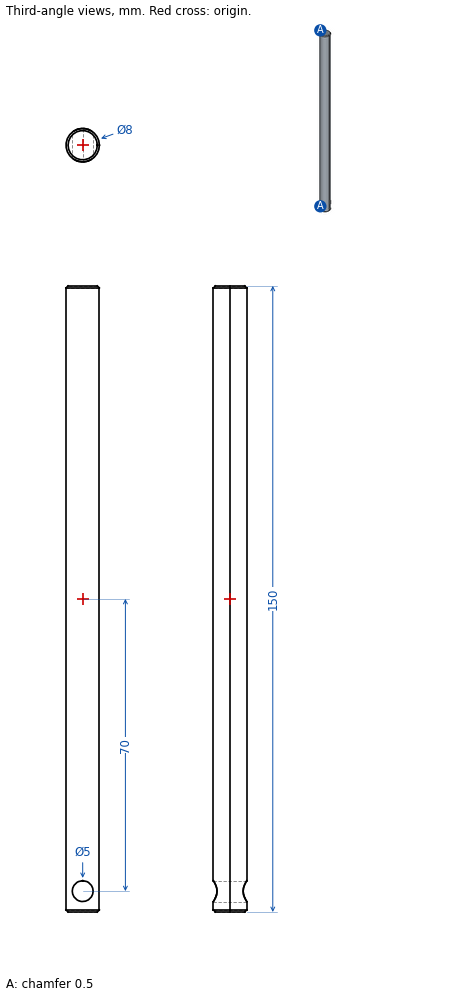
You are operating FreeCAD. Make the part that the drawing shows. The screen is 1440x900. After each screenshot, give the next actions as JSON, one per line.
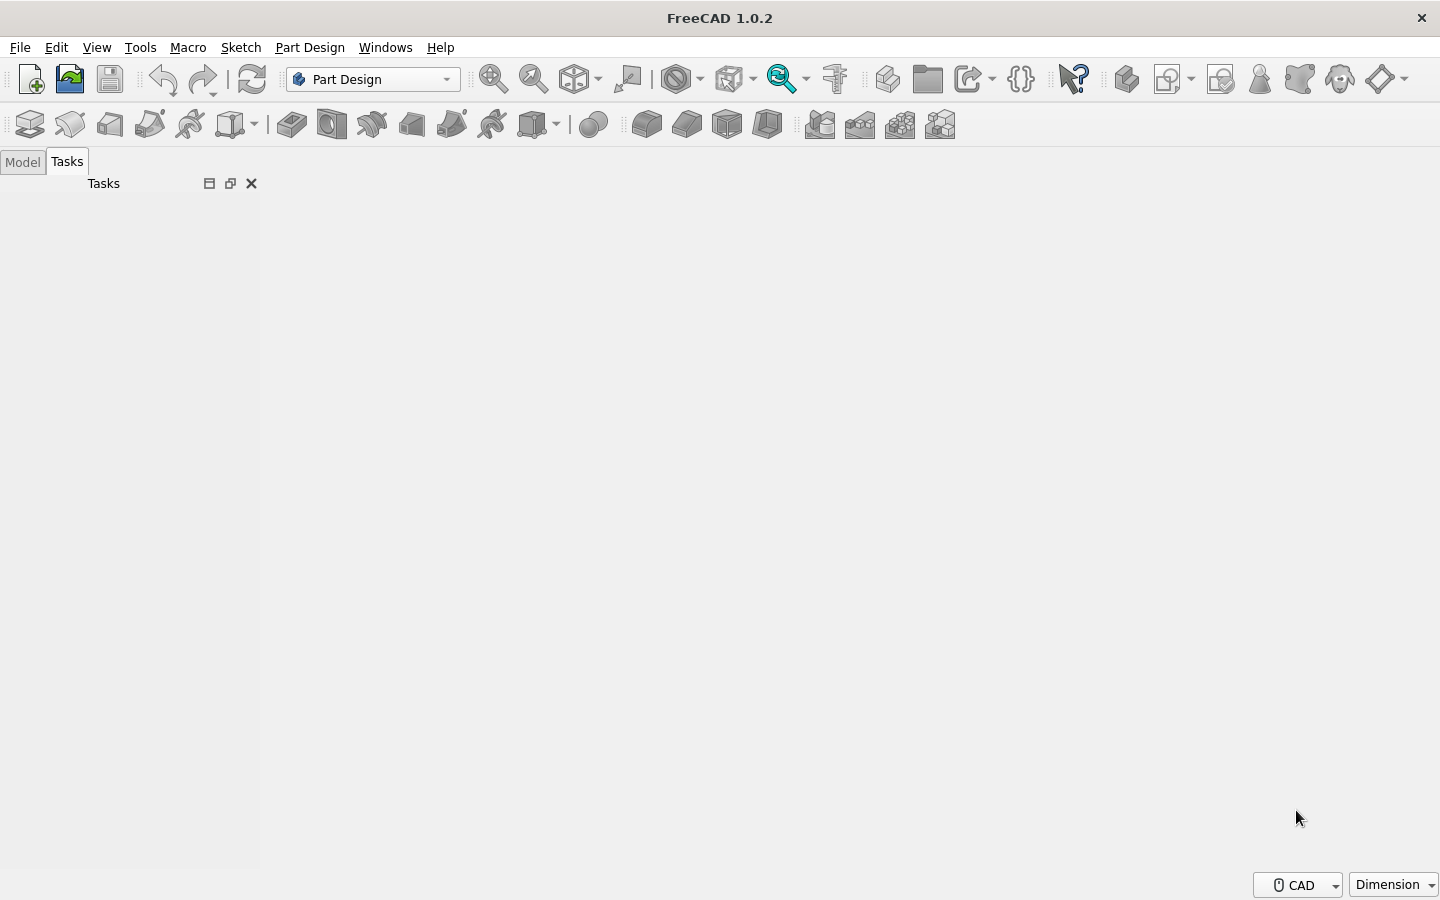
{"action": "key", "text": "ctrl+n"}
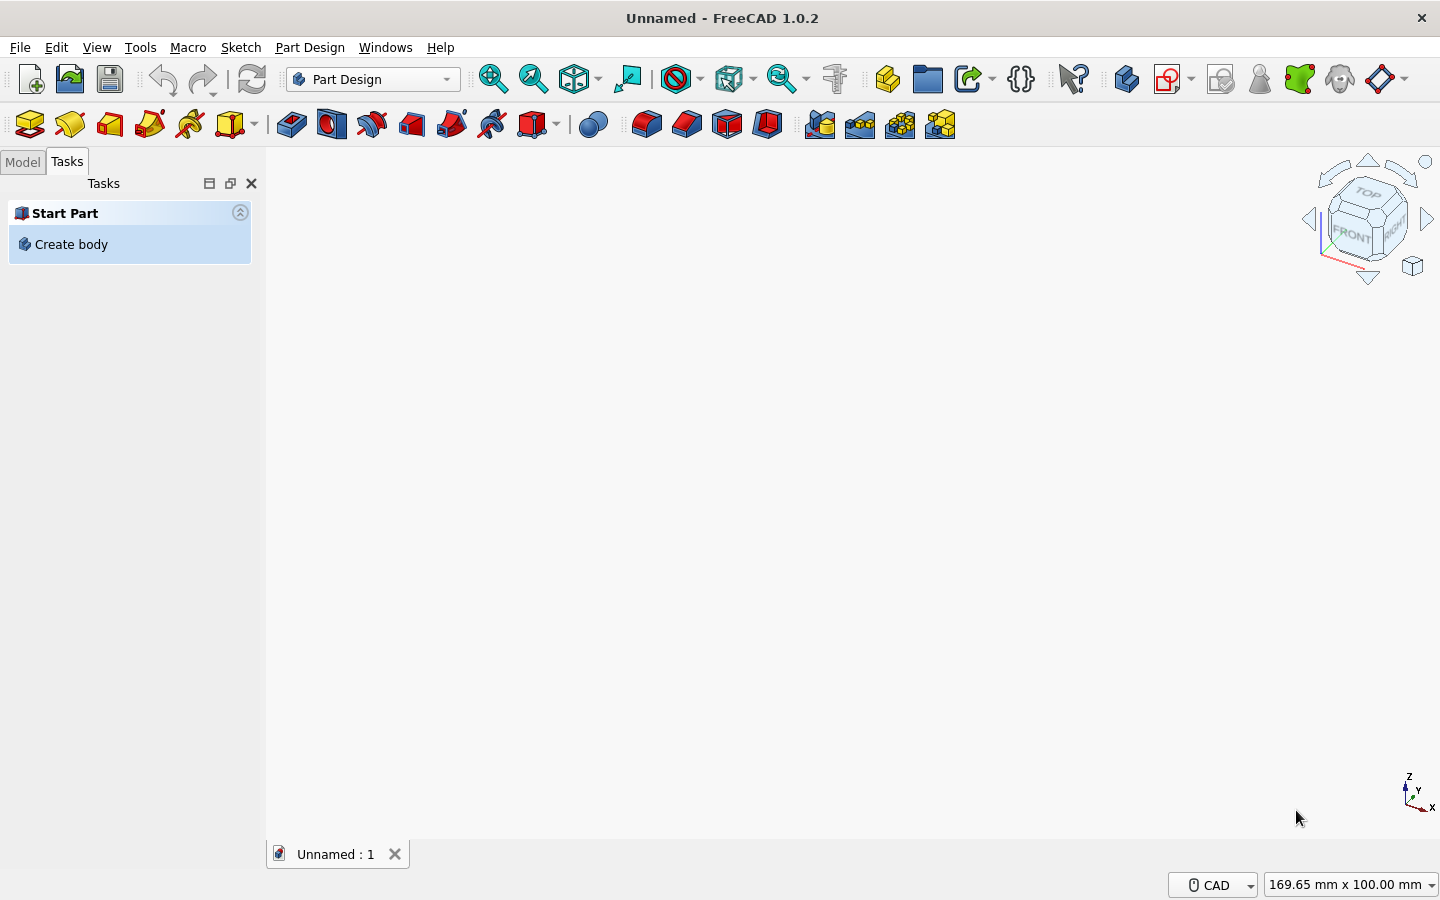
{"action": "left_click", "coordinate": [1168, 80]}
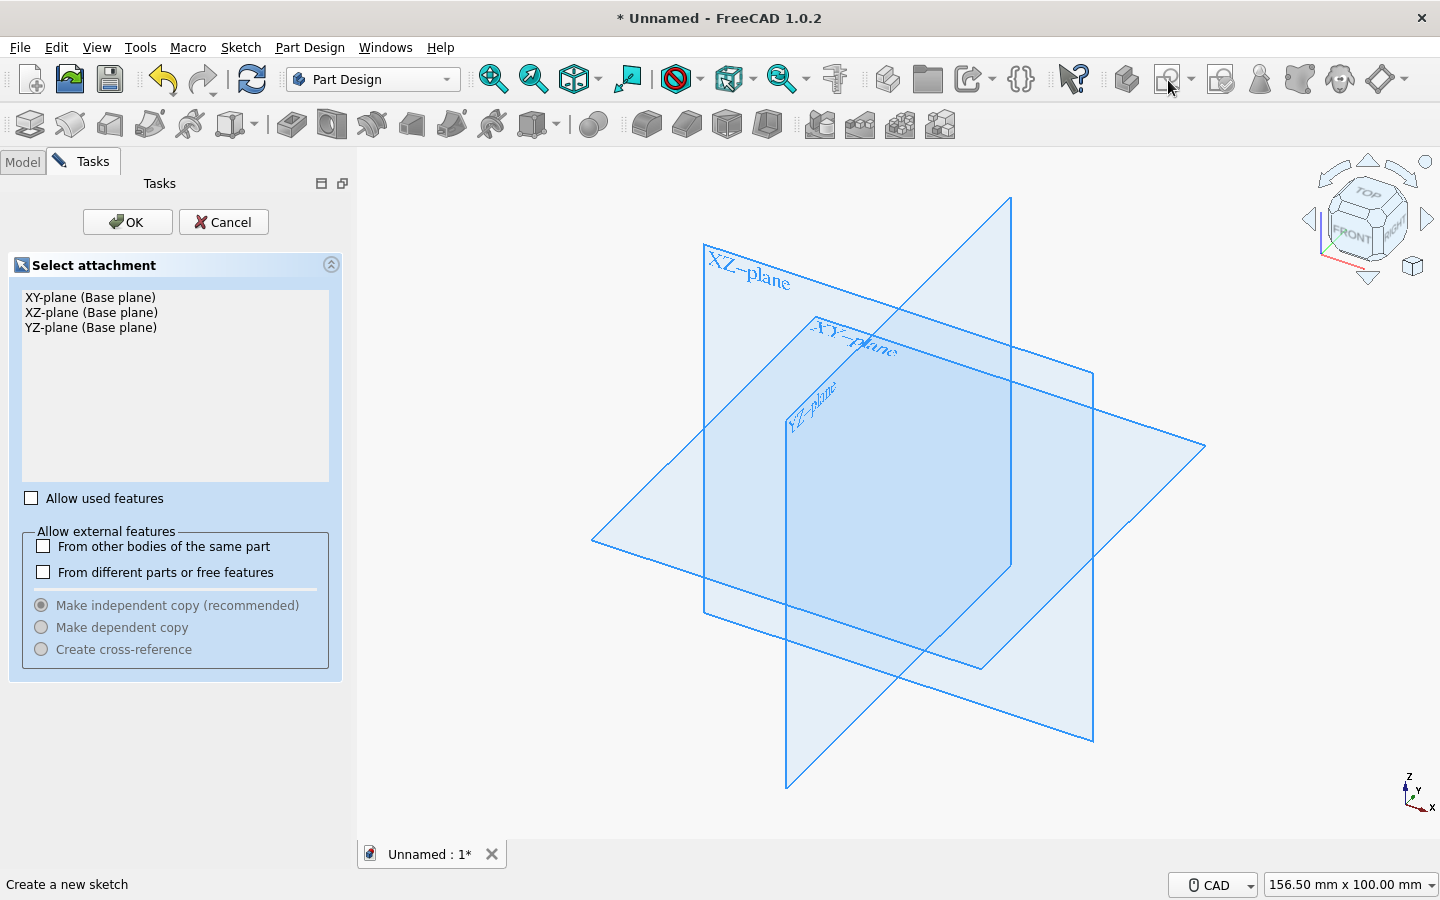
{"action": "left_click", "coordinate": [82, 298]}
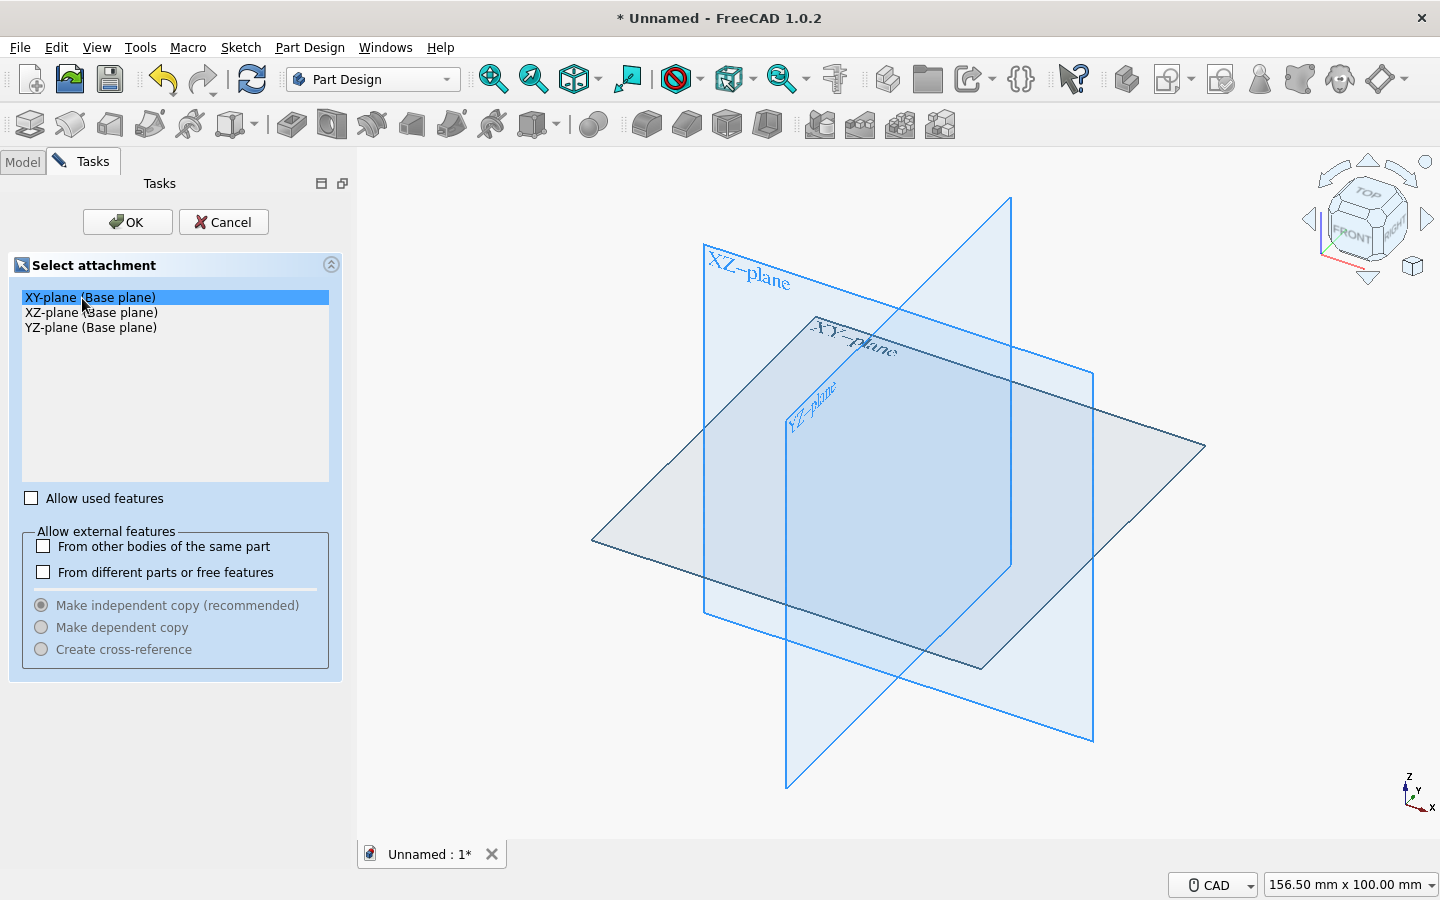
{"action": "left_click", "coordinate": [128, 222]}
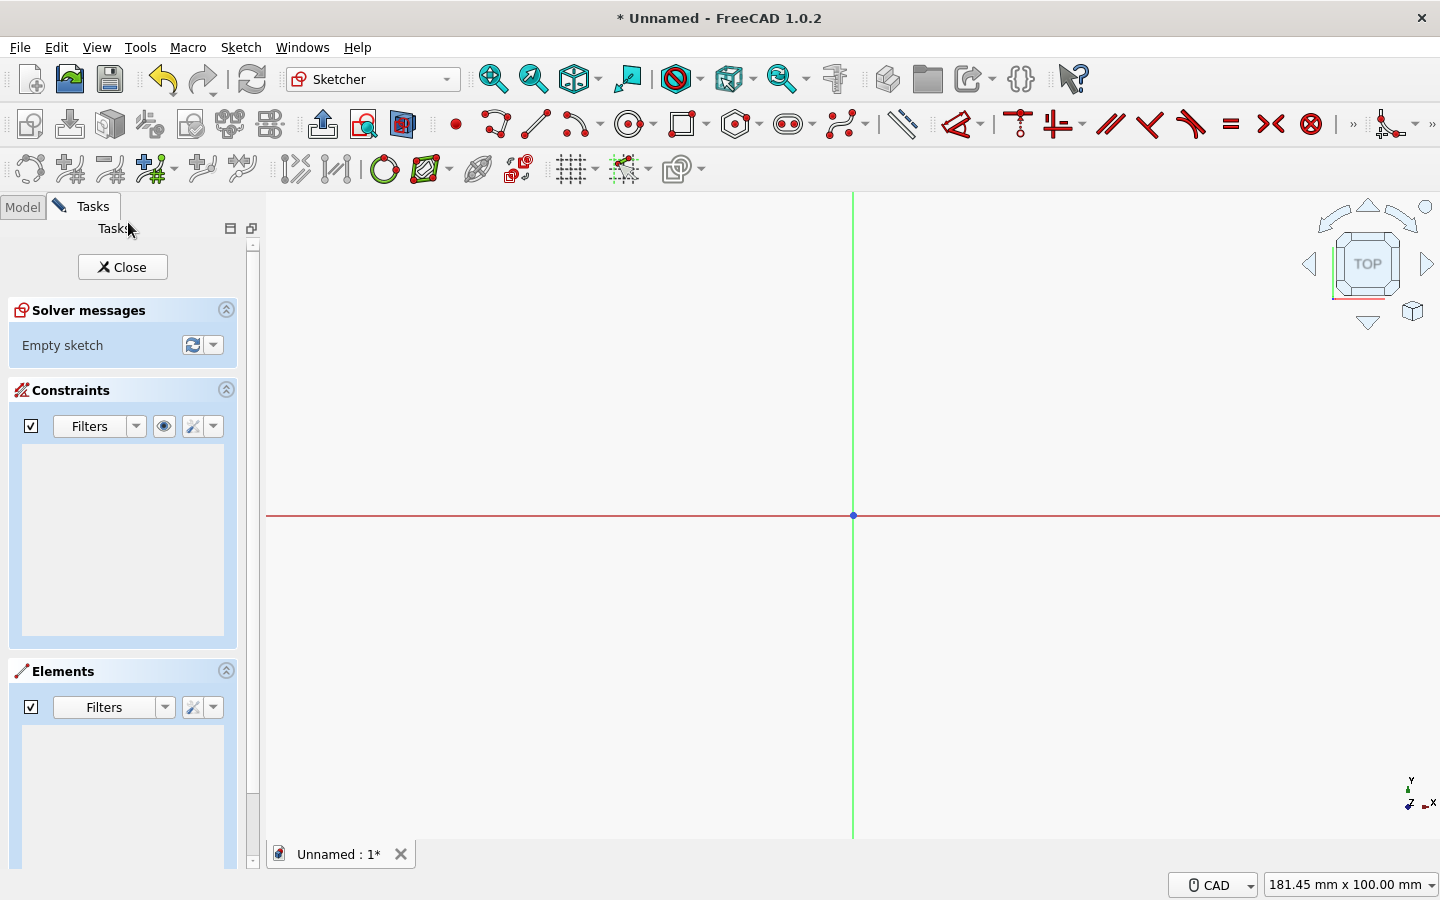
{"action": "scroll", "coordinate": [864, 516], "scroll_direction": "up", "scroll_amount": 10}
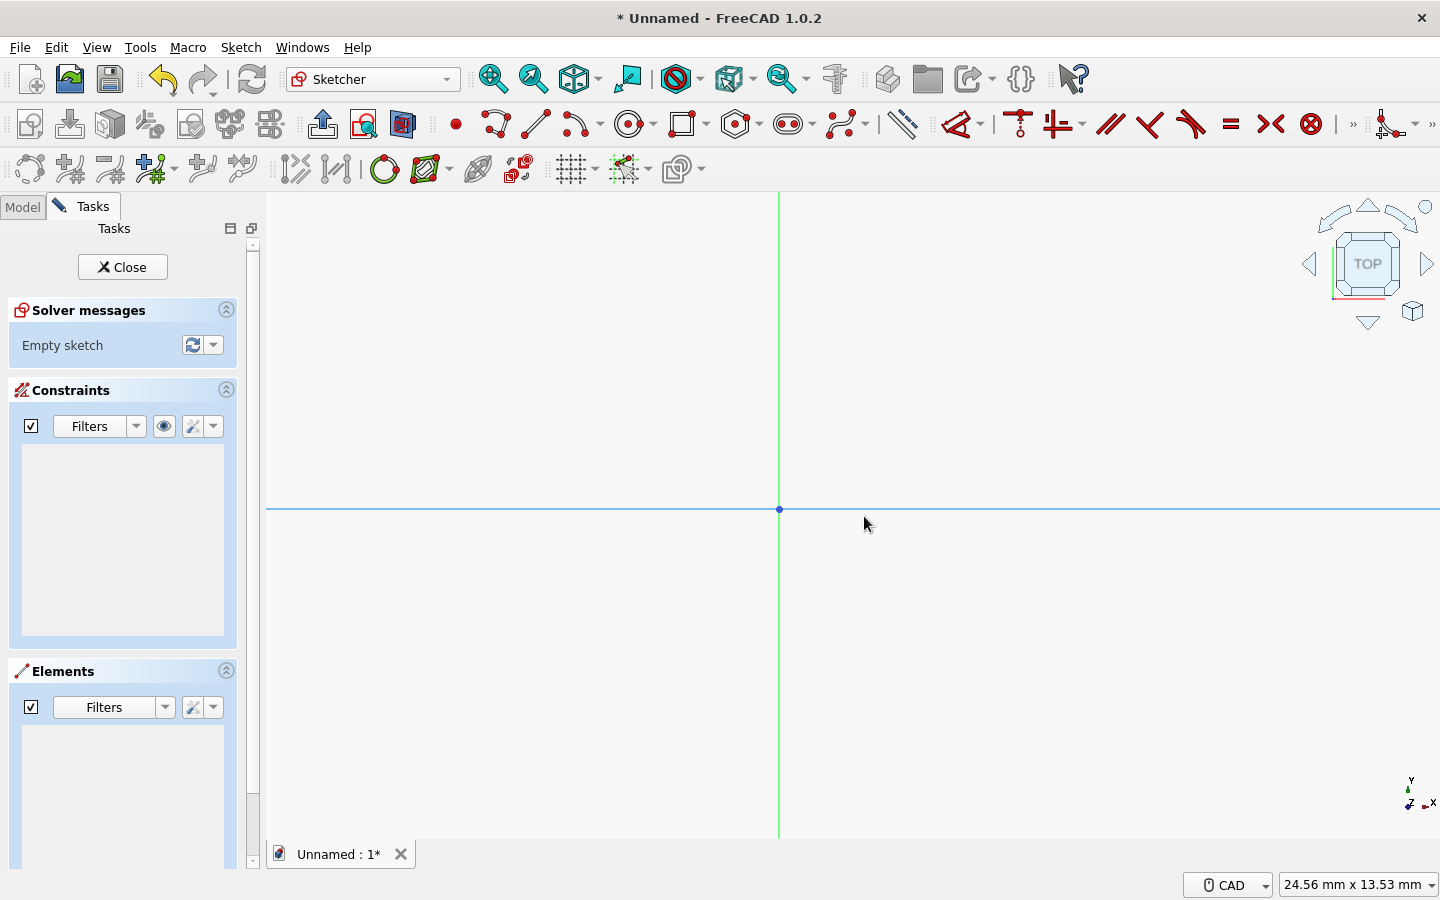
{"action": "key", "text": "g c"}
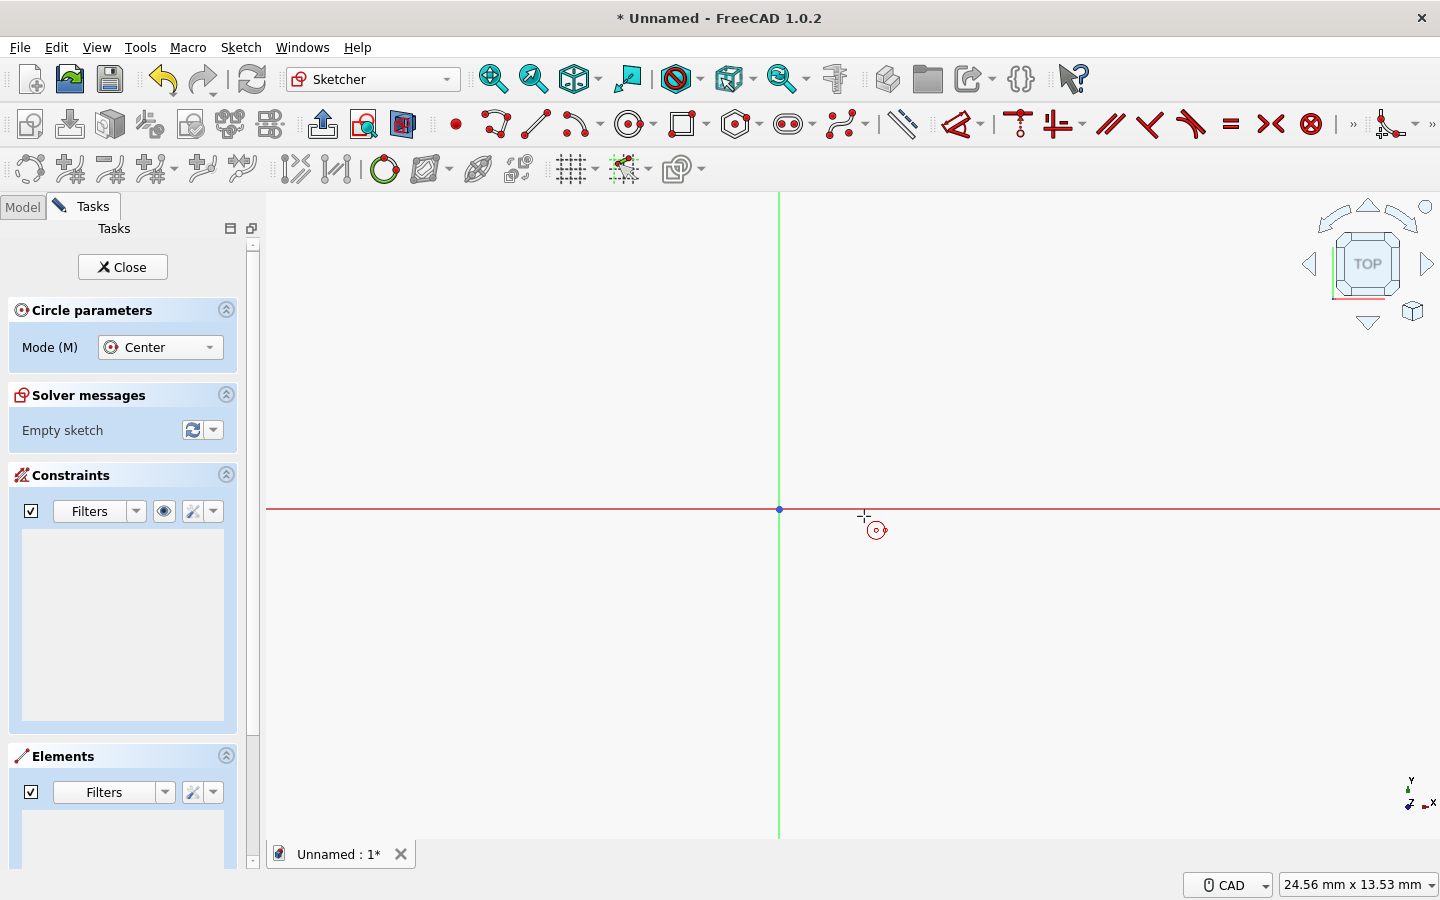
{"action": "left_click", "coordinate": [779, 509]}
{"action": "left_click", "coordinate": [915, 374]}
{"action": "key", "text": "Escape"}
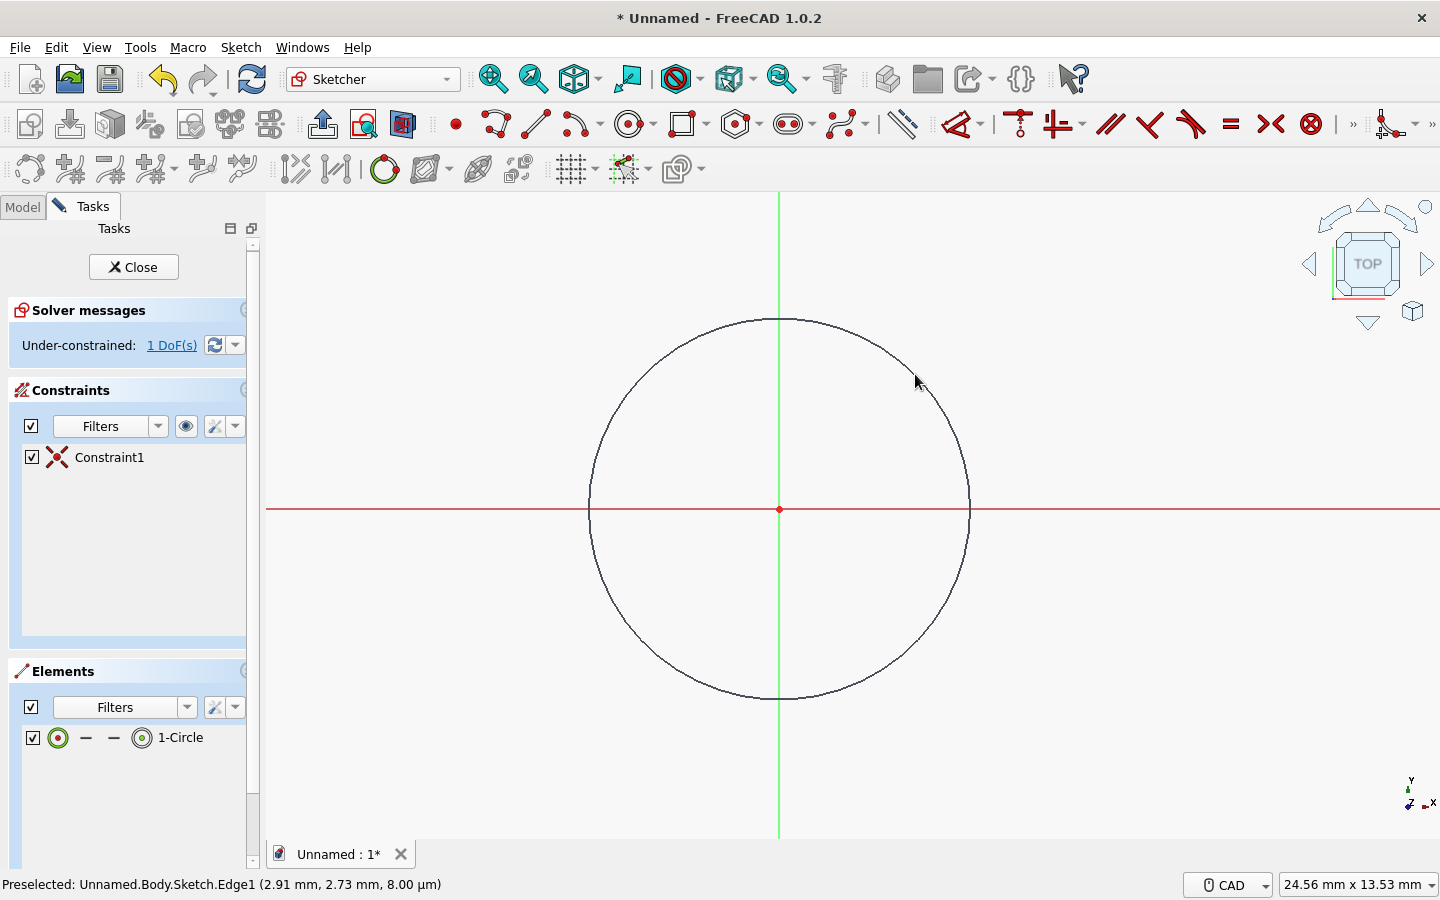
{"action": "key", "text": "d"}